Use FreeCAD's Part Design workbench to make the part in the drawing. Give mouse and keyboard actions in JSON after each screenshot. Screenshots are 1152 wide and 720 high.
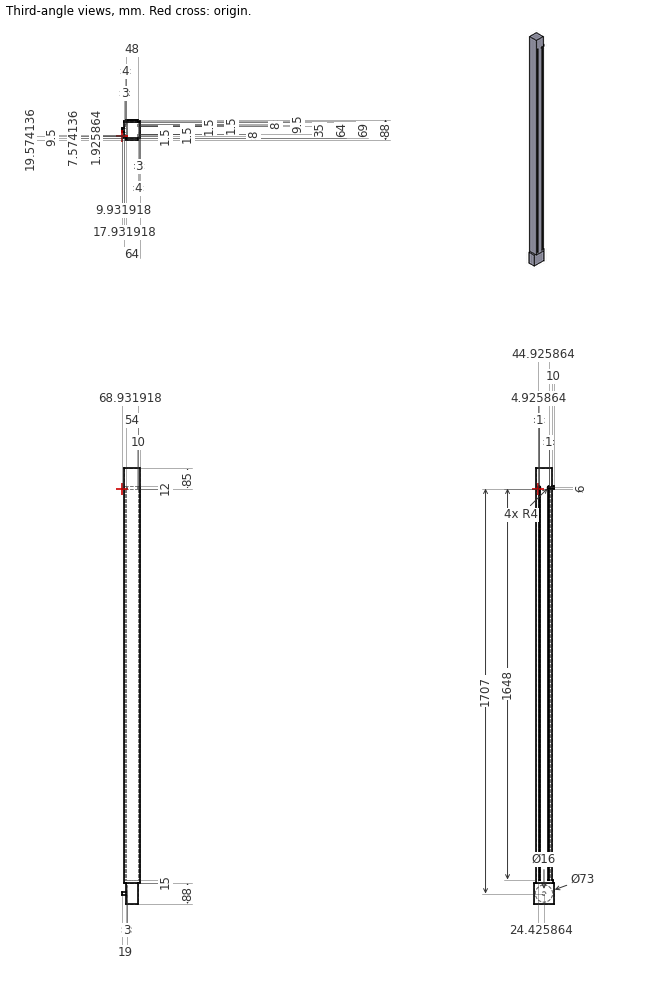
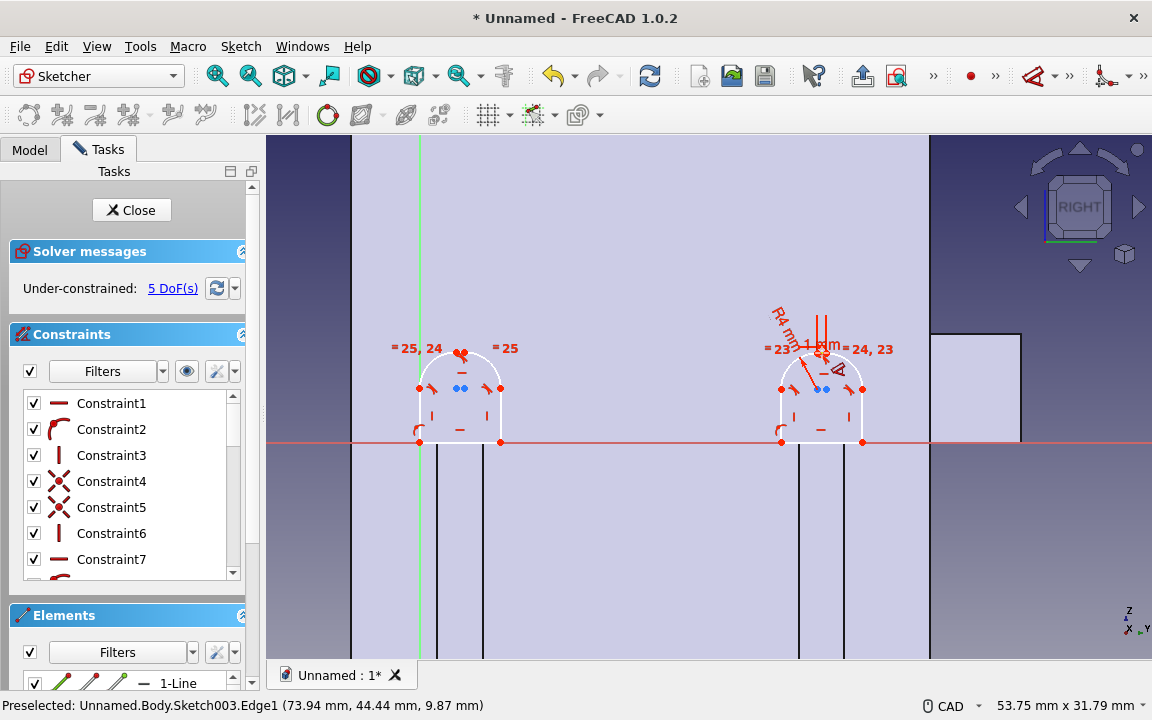
{"action": "left_click", "coordinate": [781, 406]}
{"action": "left_click", "coordinate": [815, 416]}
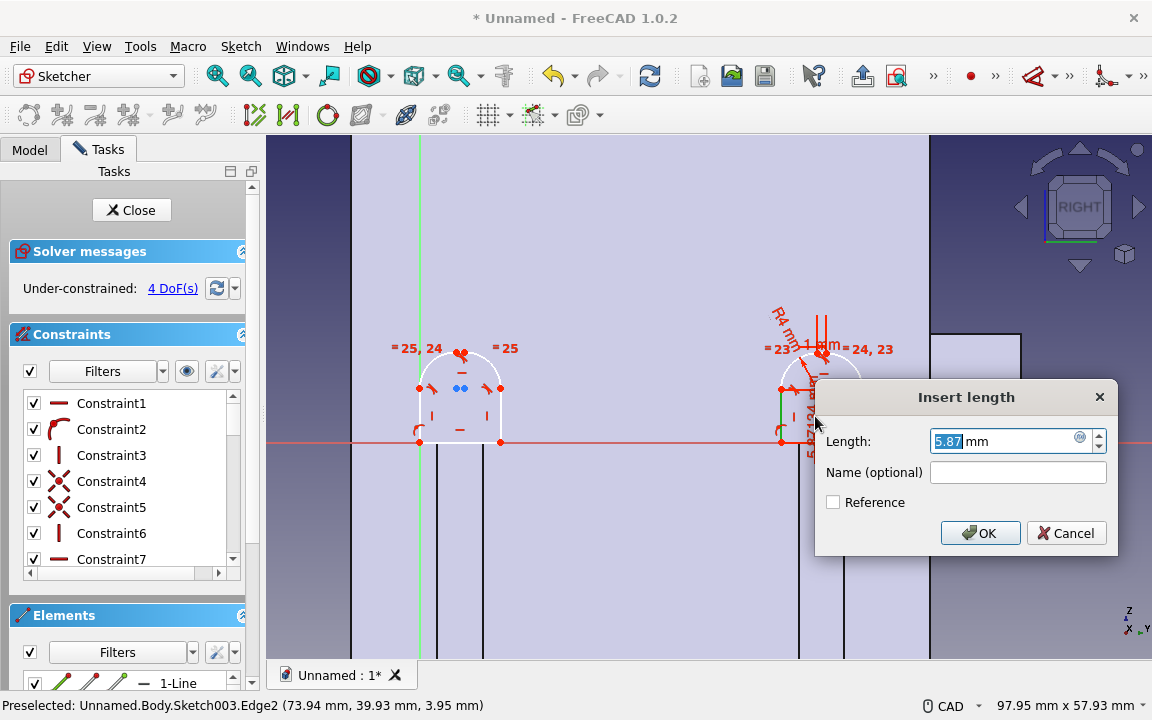
{"action": "type", "text": "6"}
{"action": "key", "text": "Return"}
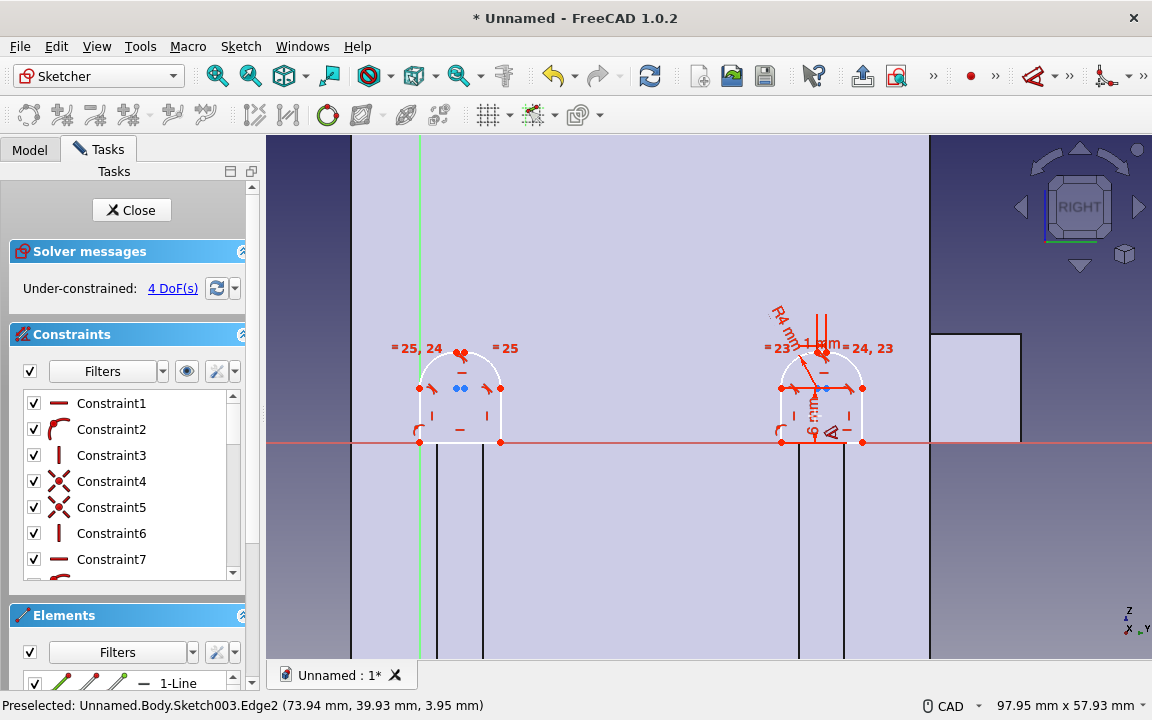
{"action": "scroll", "coordinate": [460, 352], "scroll_direction": "up", "scroll_amount": 8}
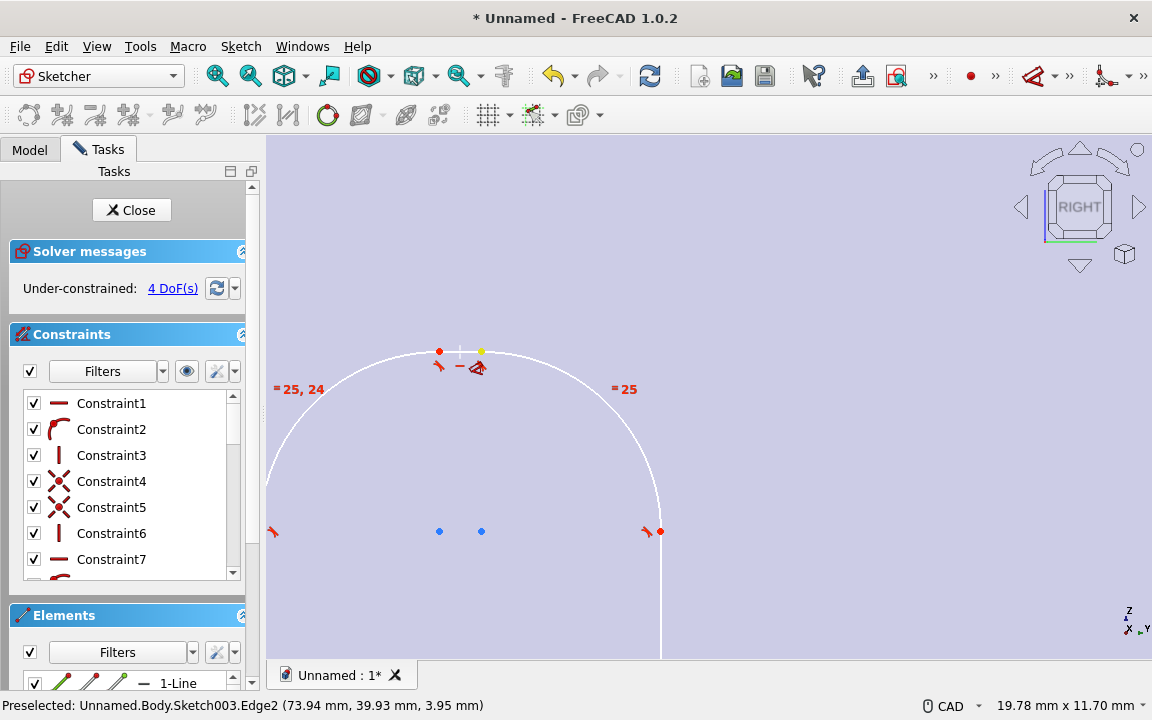
{"action": "left_click", "coordinate": [461, 352]}
{"action": "left_click", "coordinate": [461, 318]}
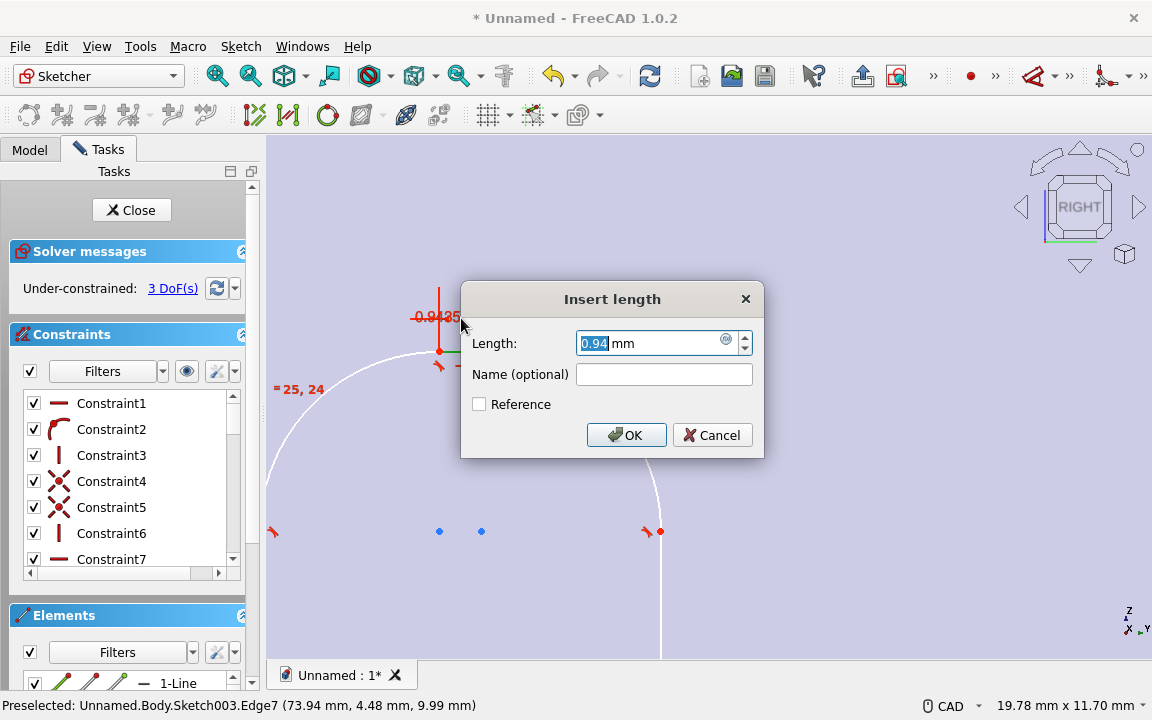
{"action": "type", "text": "1"}
{"action": "key", "text": "Return"}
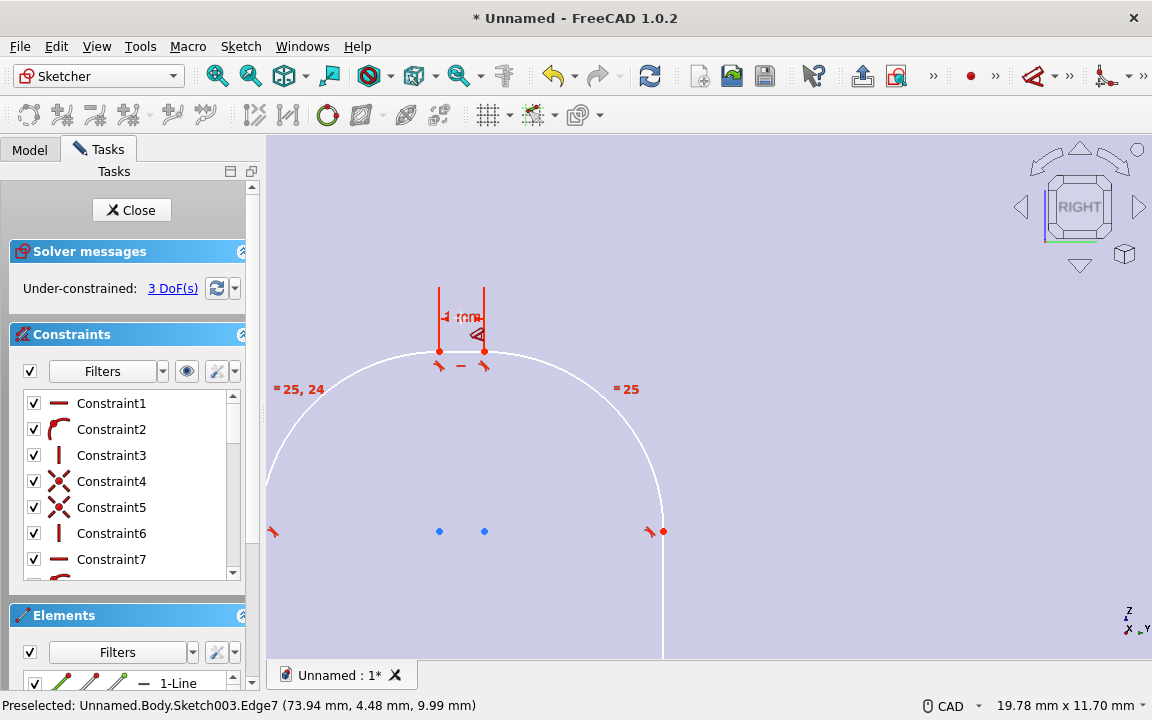
{"action": "scroll", "coordinate": [460, 352], "scroll_direction": "down", "scroll_amount": 8}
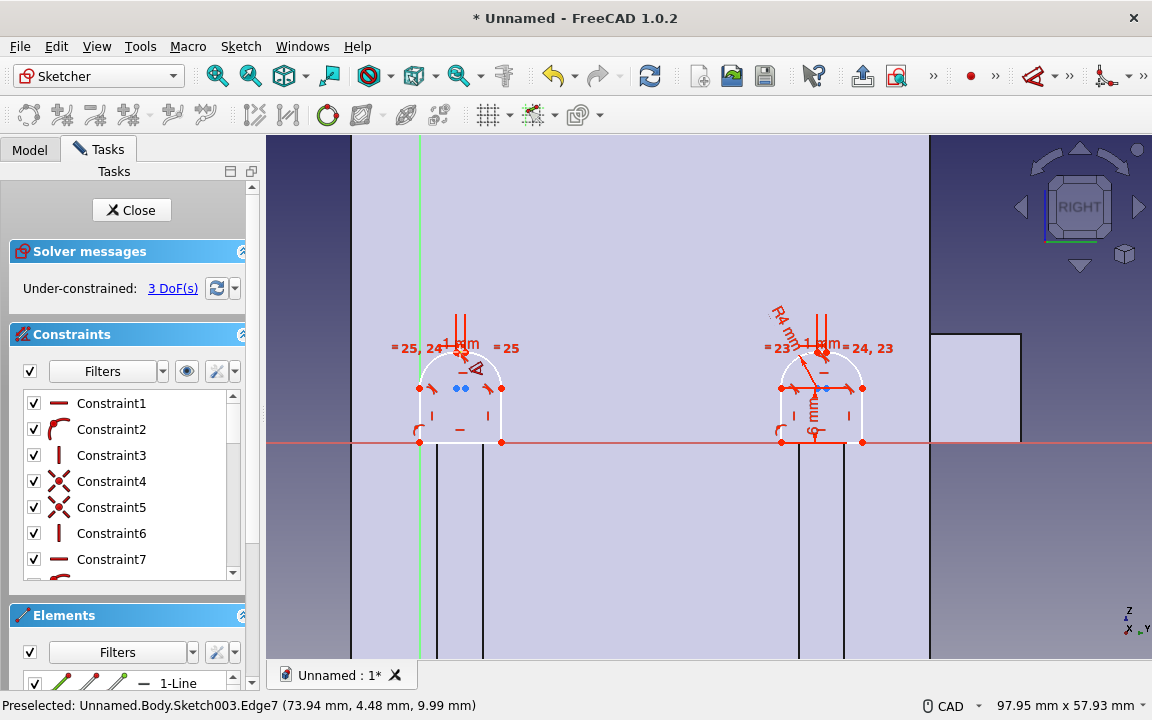
{"action": "left_click", "coordinate": [420, 405]}
{"action": "left_click", "coordinate": [386, 416]}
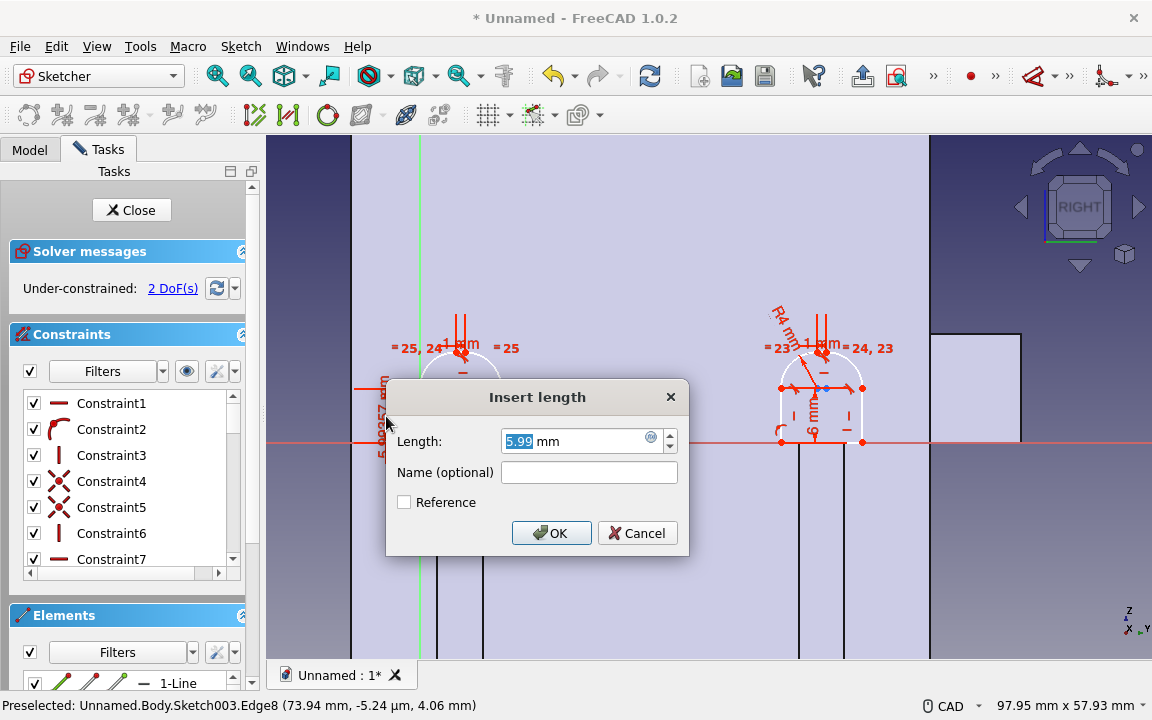
{"action": "type", "text": "6"}
{"action": "key", "text": "Return"}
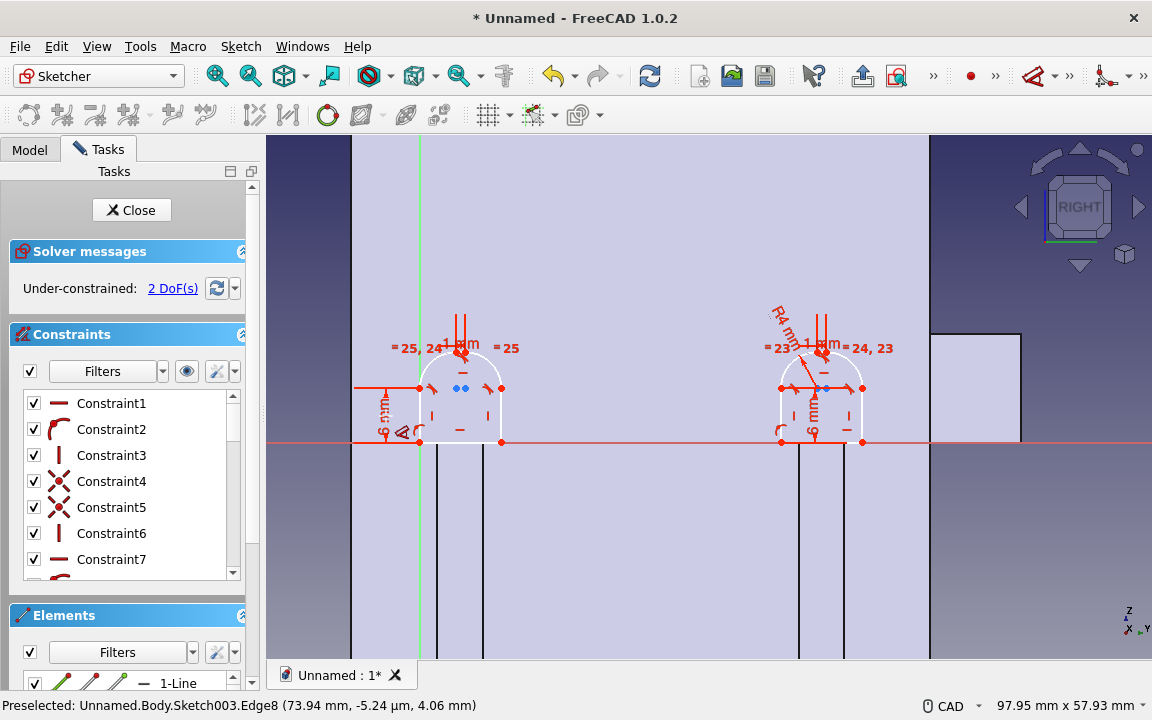
{"action": "scroll", "coordinate": [465, 352], "scroll_direction": "up", "scroll_amount": 2}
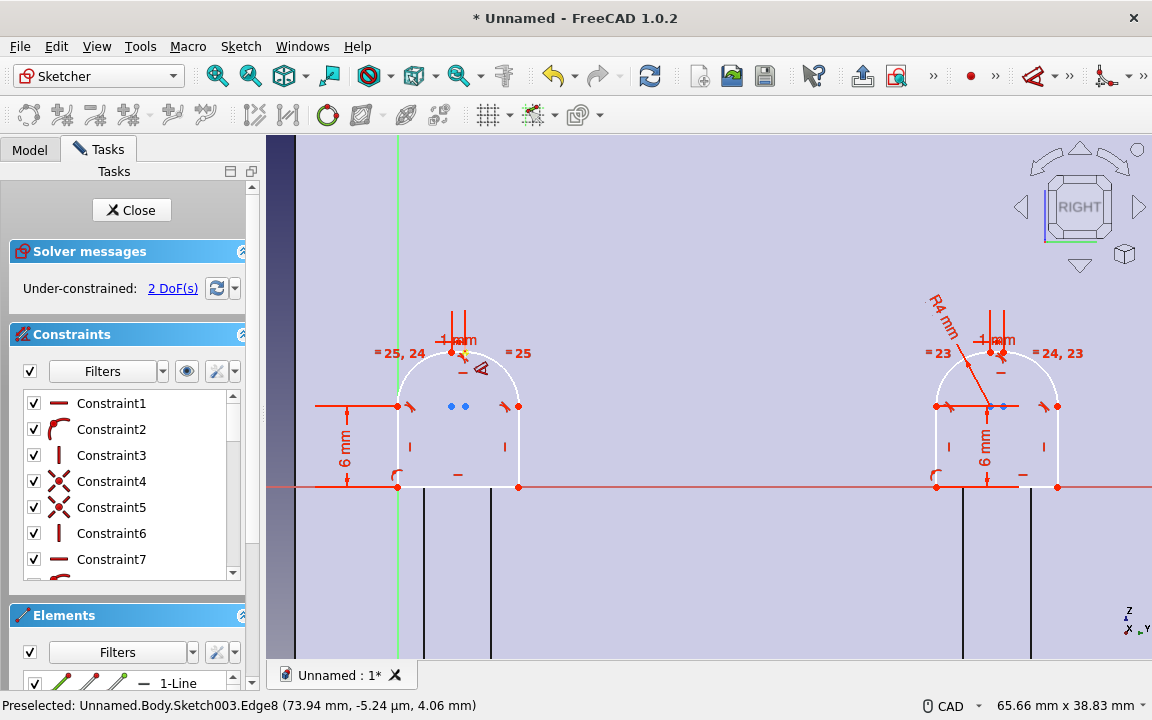
{"action": "left_click", "coordinate": [465, 352]}
{"action": "left_click", "coordinate": [431, 521]}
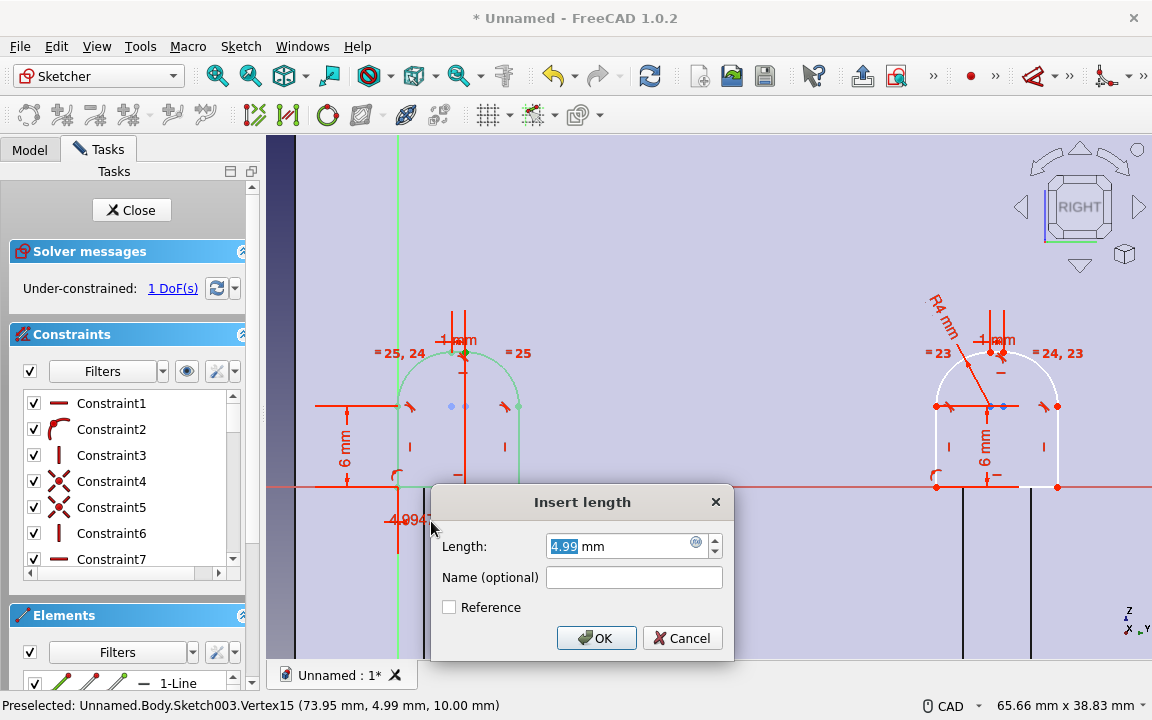
{"action": "type", "text": "4.925864"}
{"action": "key", "text": "Return"}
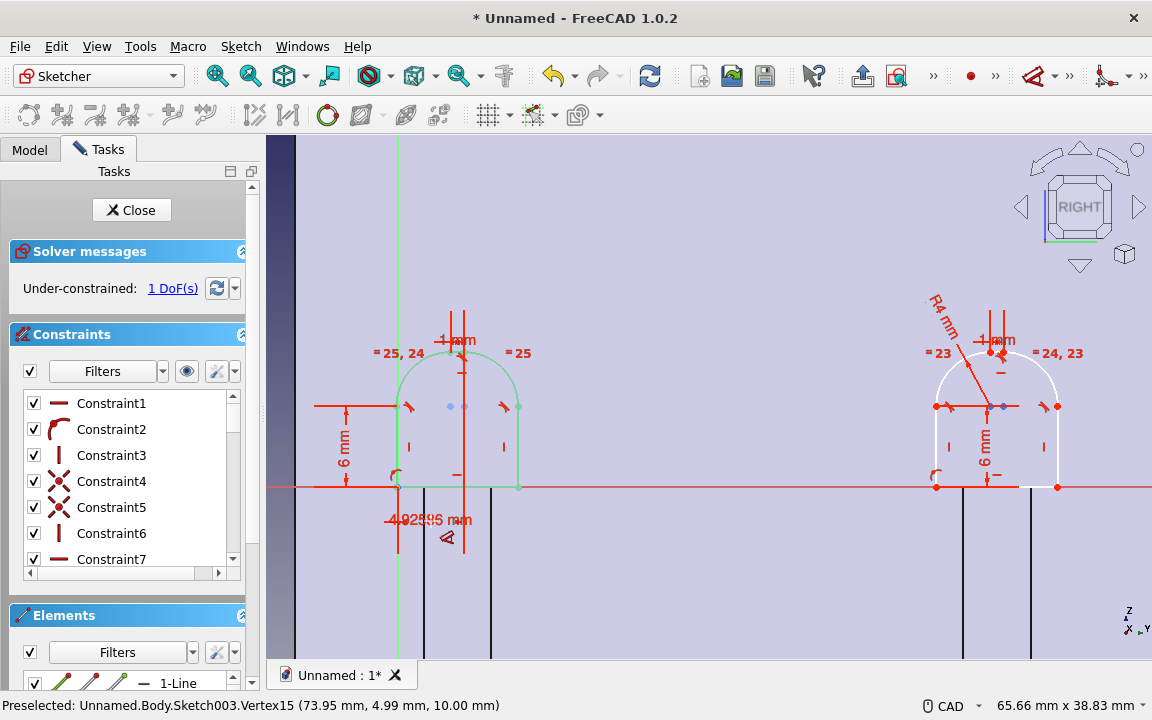
{"action": "scroll", "coordinate": [464, 351], "scroll_direction": "down", "scroll_amount": 2}